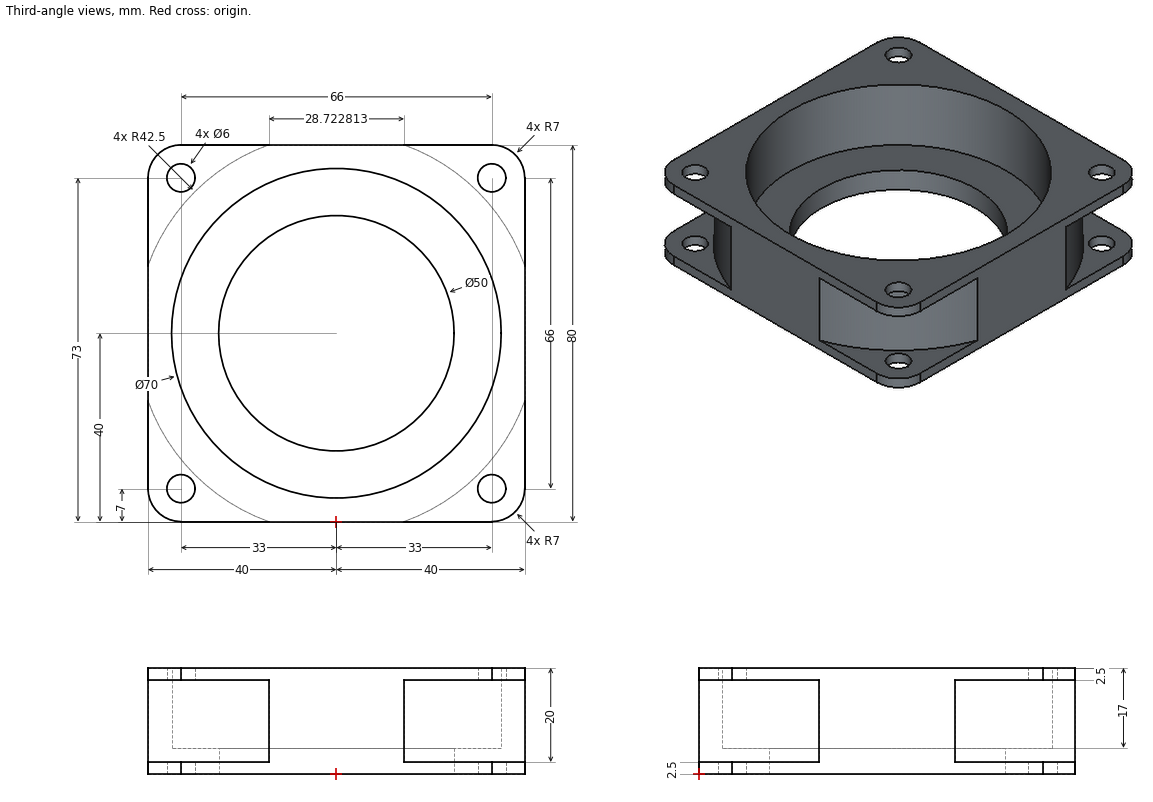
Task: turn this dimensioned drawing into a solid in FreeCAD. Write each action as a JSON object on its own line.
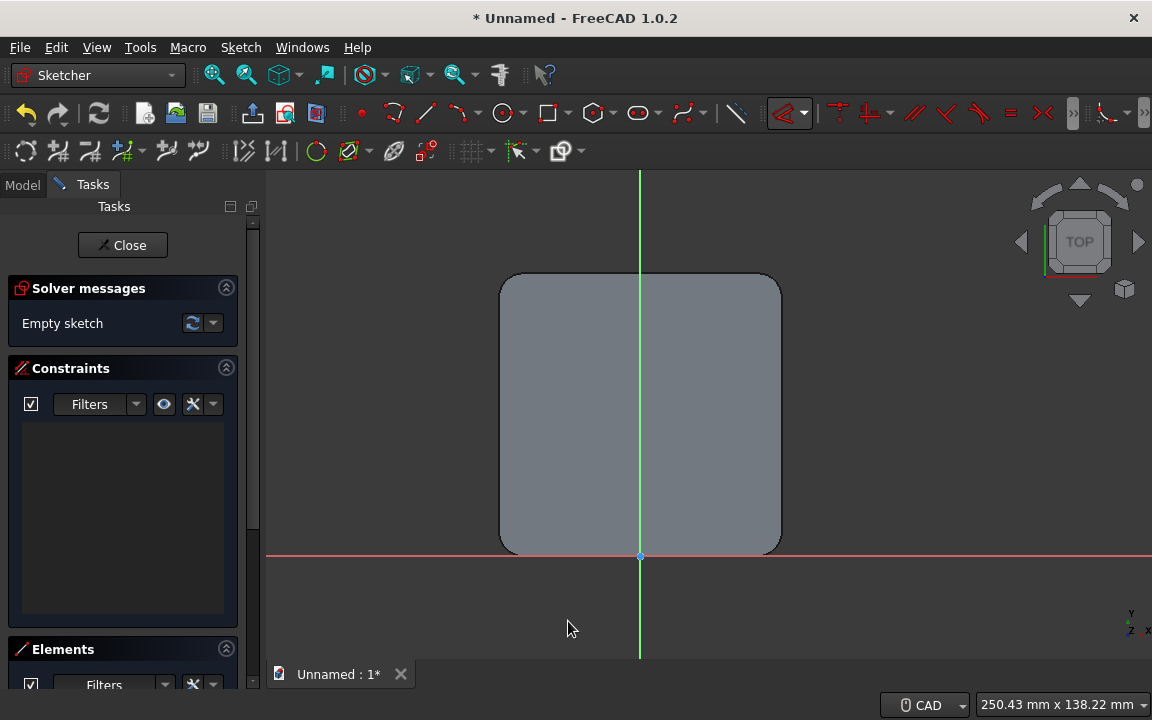
{"action": "left_click", "coordinate": [426, 114]}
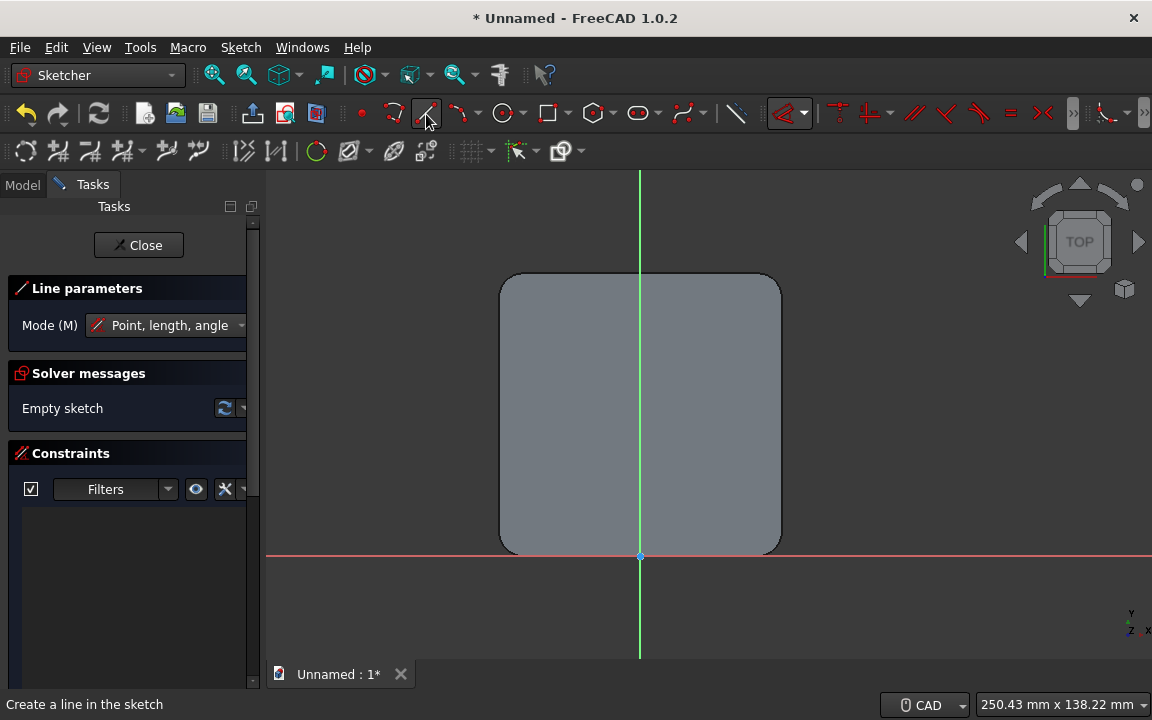
{"action": "left_click", "coordinate": [691, 273]}
{"action": "left_click", "coordinate": [590, 273]}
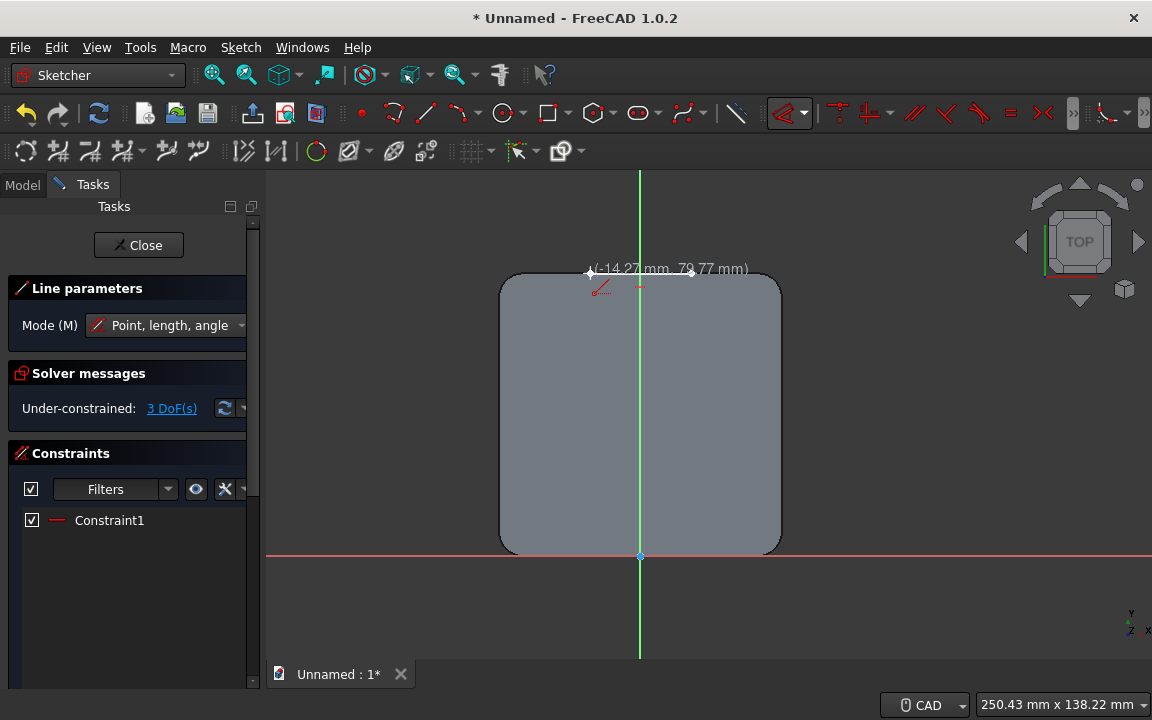
{"action": "left_click", "coordinate": [499, 364]}
{"action": "left_click", "coordinate": [499, 466]}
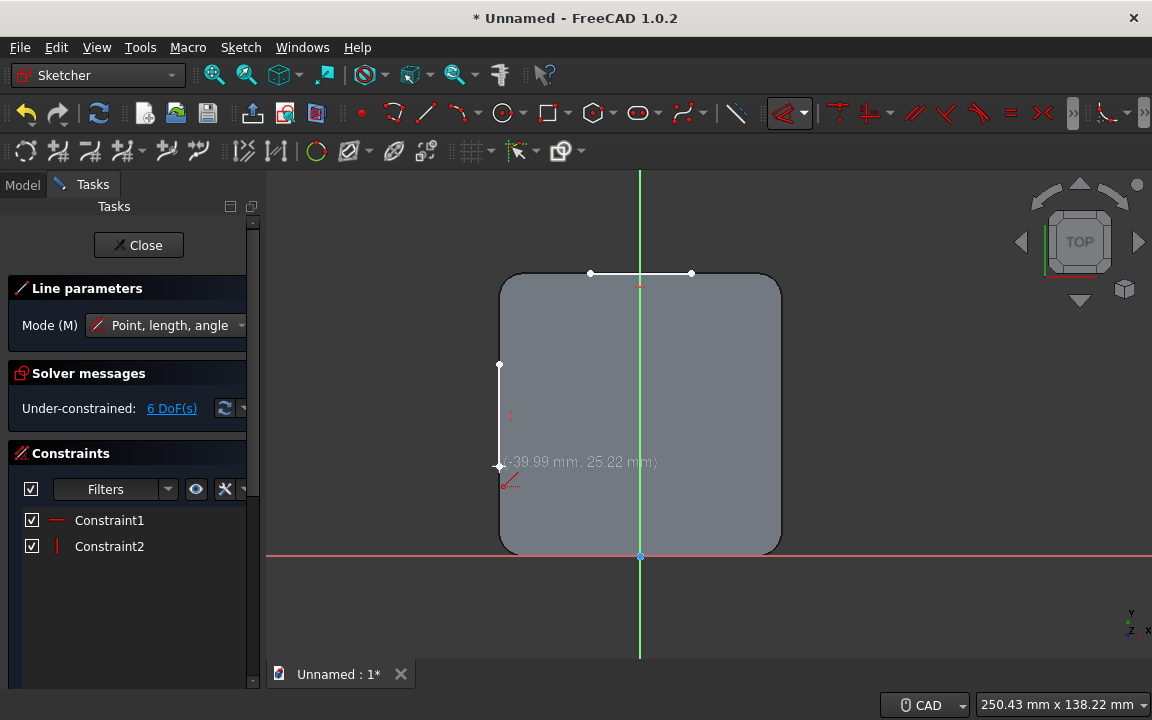
{"action": "left_click", "coordinate": [590, 556]}
{"action": "left_click", "coordinate": [691, 547]}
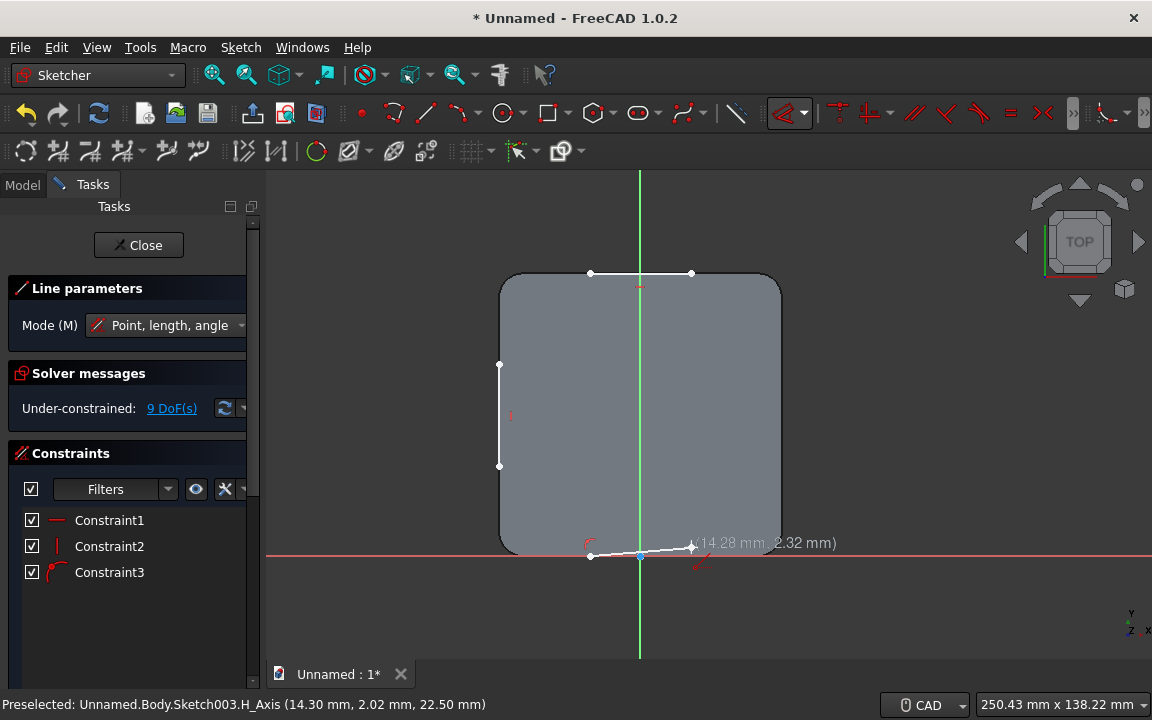
{"action": "left_click", "coordinate": [782, 466]}
{"action": "left_click", "coordinate": [782, 364]}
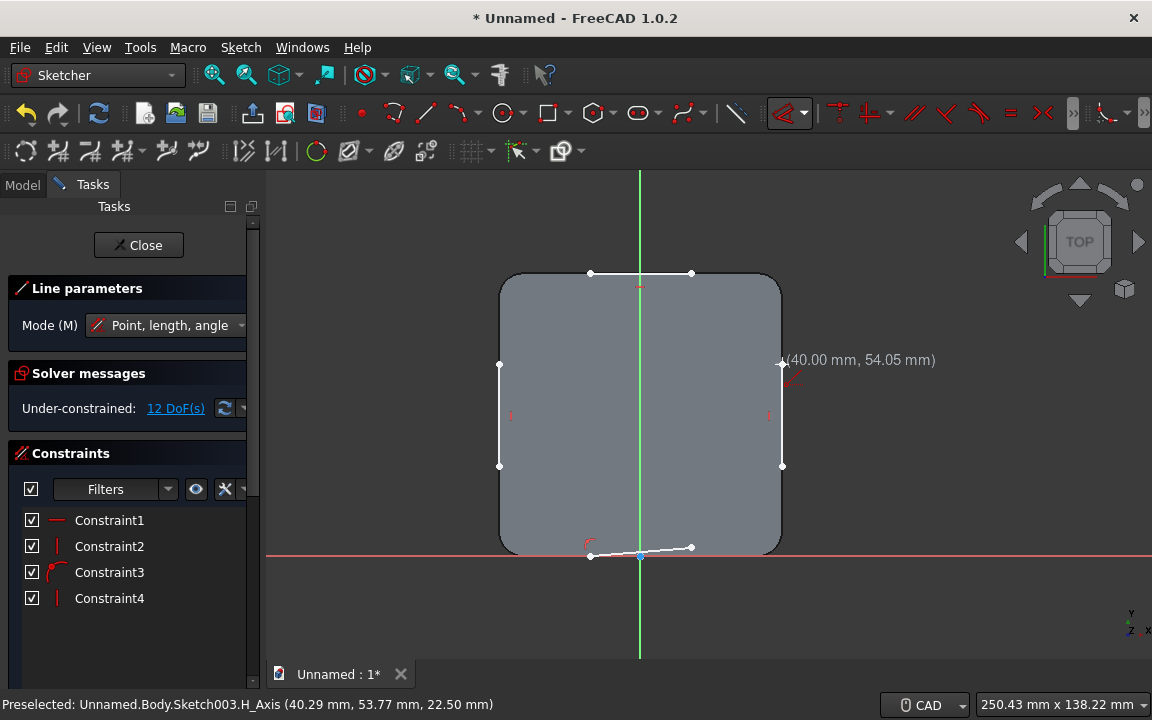
{"action": "left_click", "coordinate": [458, 114]}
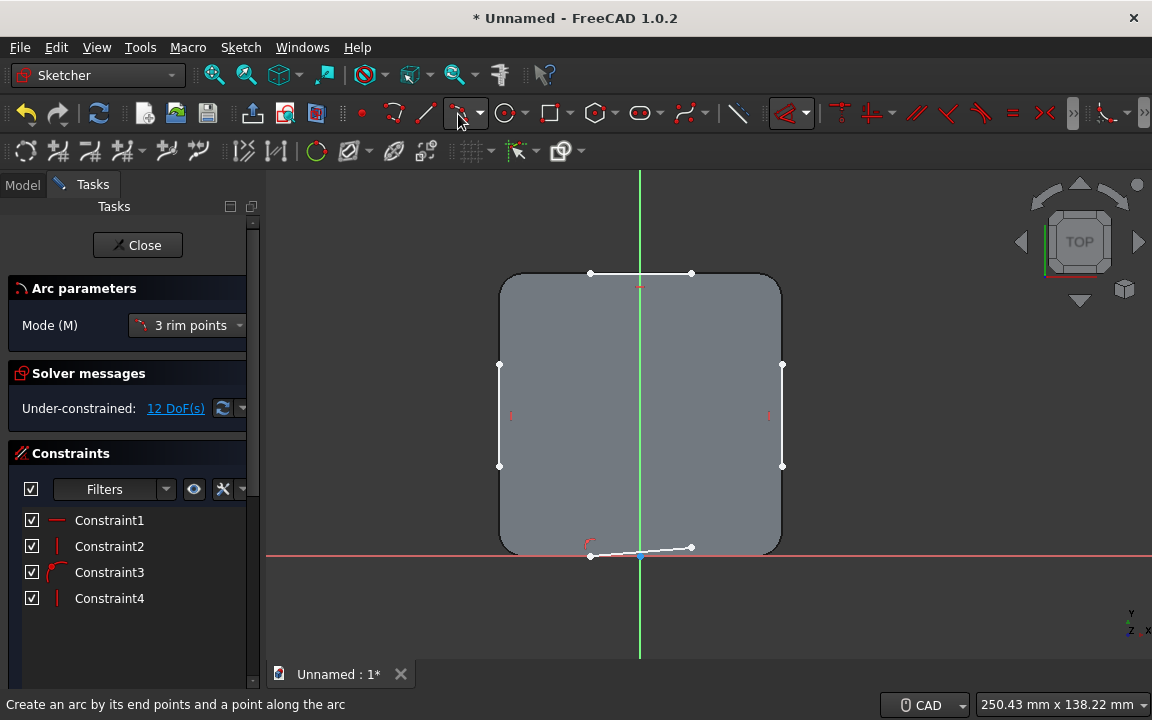
{"action": "left_click", "coordinate": [590, 274]}
{"action": "left_click", "coordinate": [499, 365]}
{"action": "left_click", "coordinate": [534, 308]}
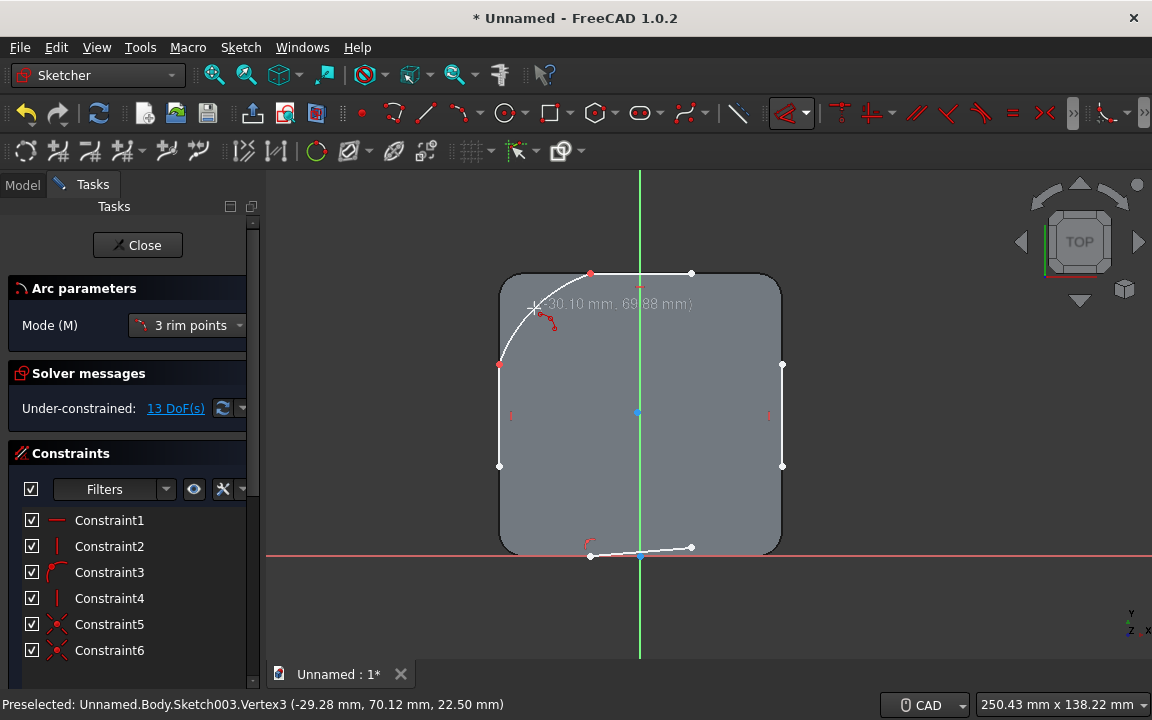
{"action": "left_click", "coordinate": [499, 467]}
{"action": "left_click", "coordinate": [590, 556]}
{"action": "left_click", "coordinate": [534, 521]}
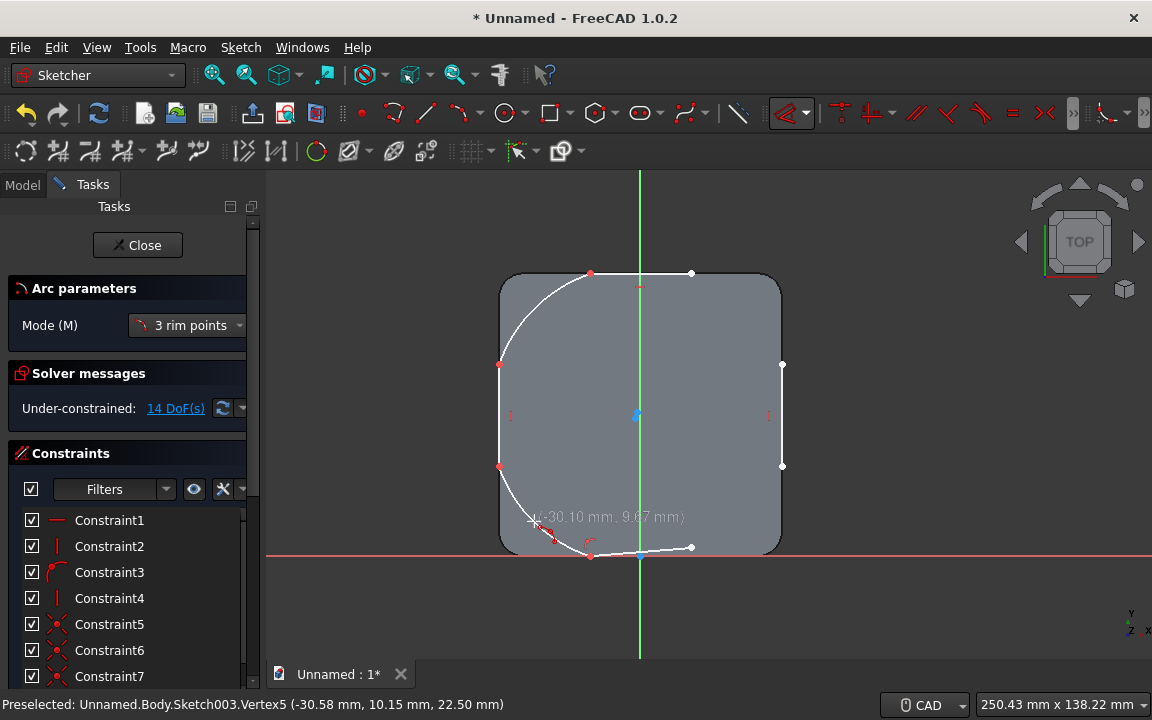
{"action": "left_click", "coordinate": [691, 548]}
{"action": "left_click", "coordinate": [782, 467]}
{"action": "left_click", "coordinate": [747, 521]}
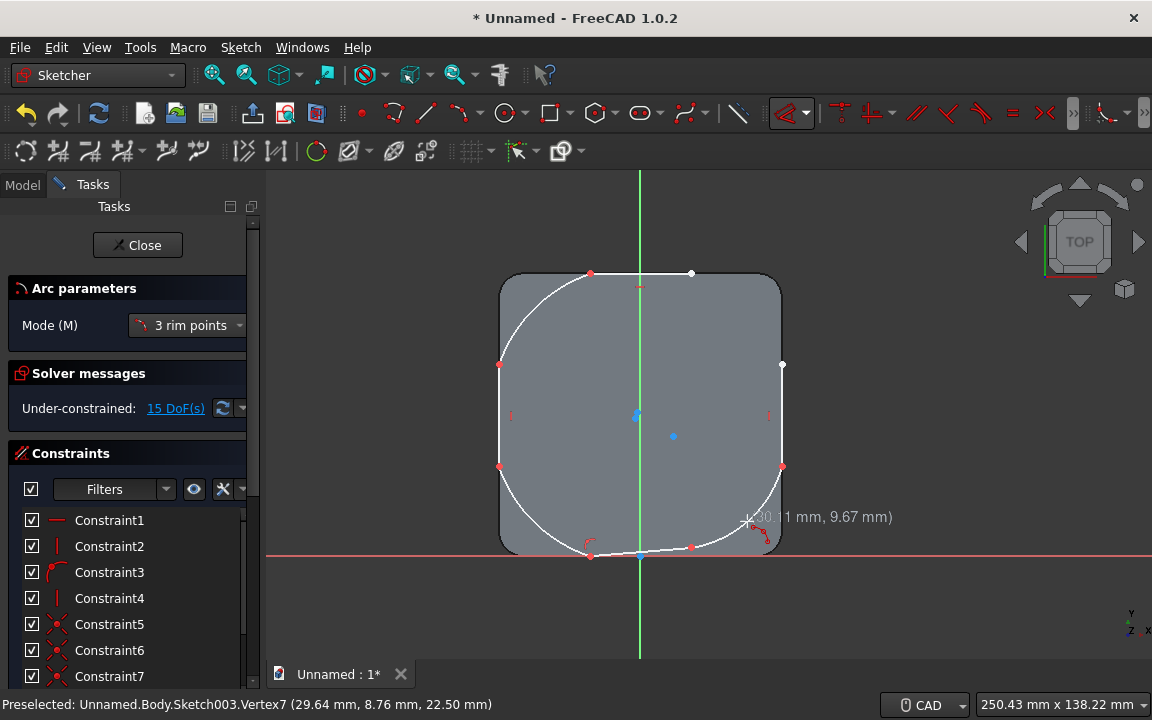
{"action": "left_click", "coordinate": [782, 365]}
{"action": "left_click", "coordinate": [691, 274]}
{"action": "left_click", "coordinate": [747, 308]}
{"action": "key", "text": "Escape"}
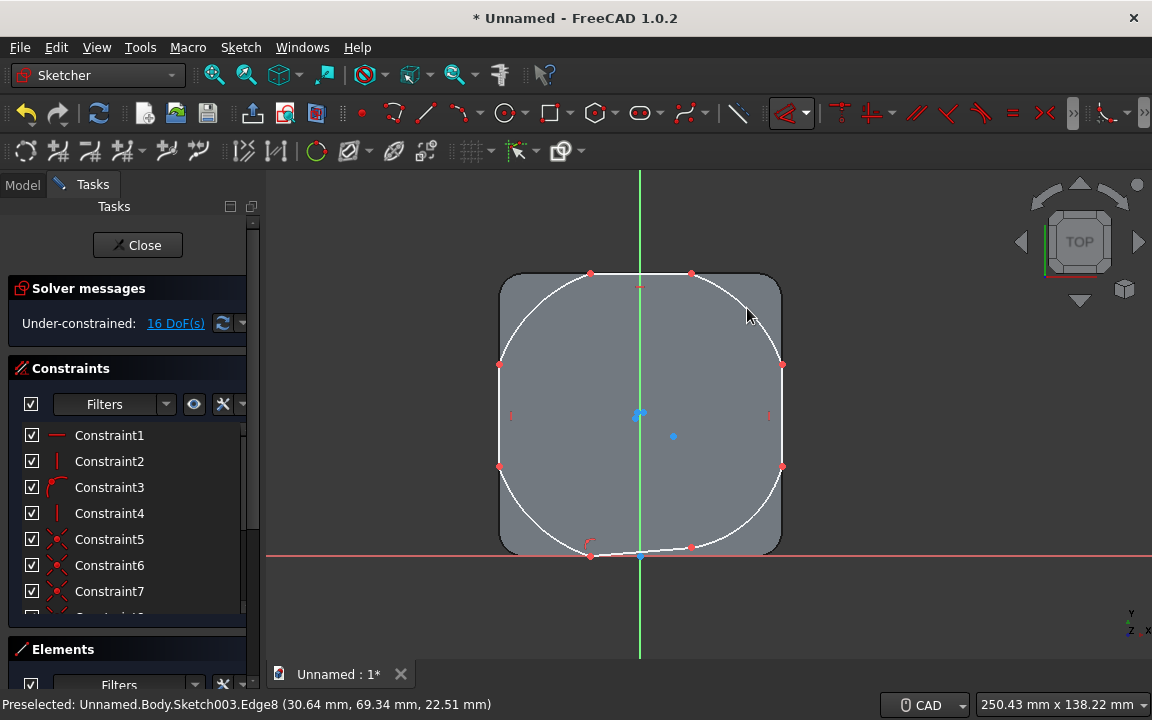
{"action": "left_click", "coordinate": [620, 554]}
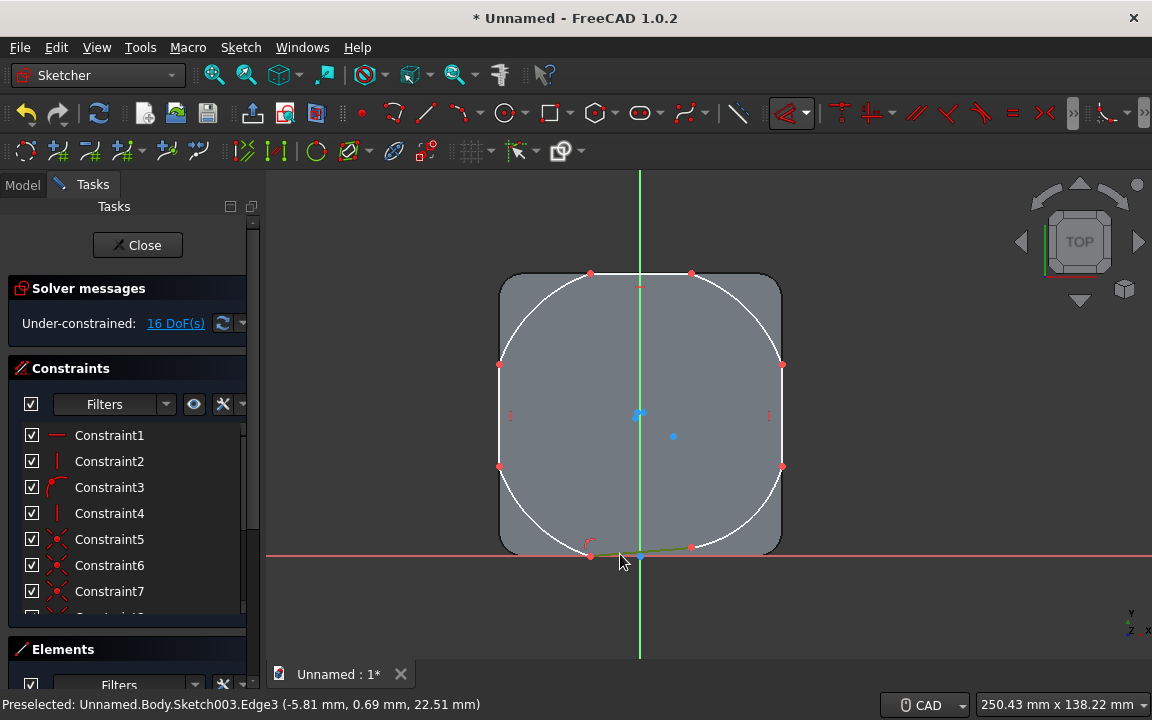
{"action": "left_click", "coordinate": [894, 114]}